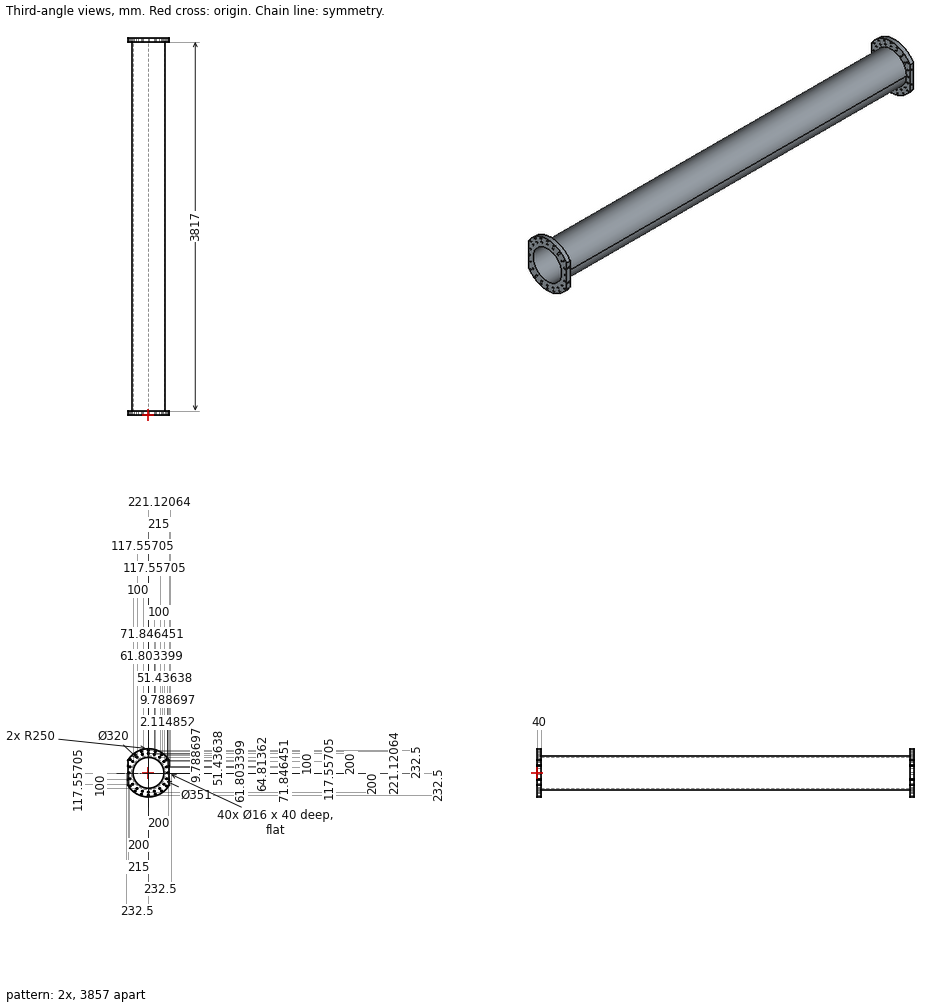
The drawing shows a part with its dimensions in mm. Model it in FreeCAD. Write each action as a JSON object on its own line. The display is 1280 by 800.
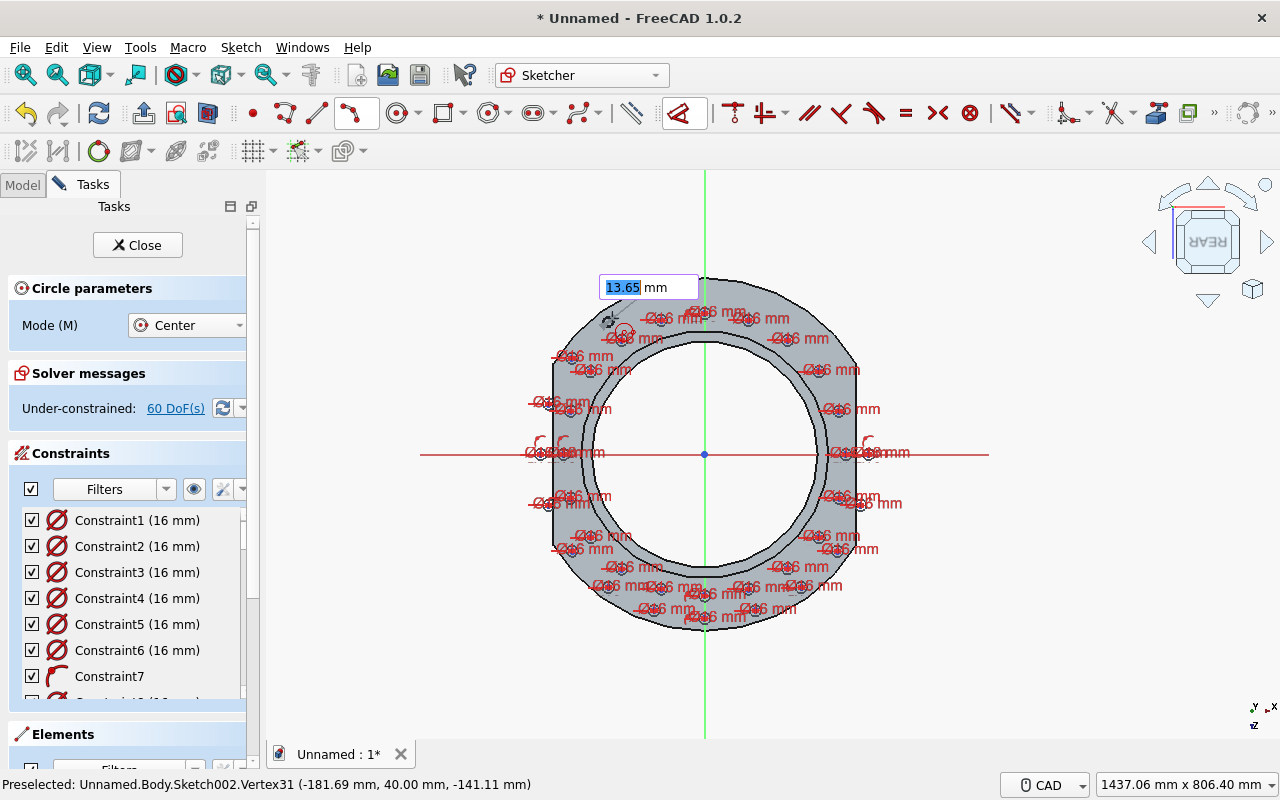
{"action": "type", "text": "16"}
{"action": "key", "text": "Return"}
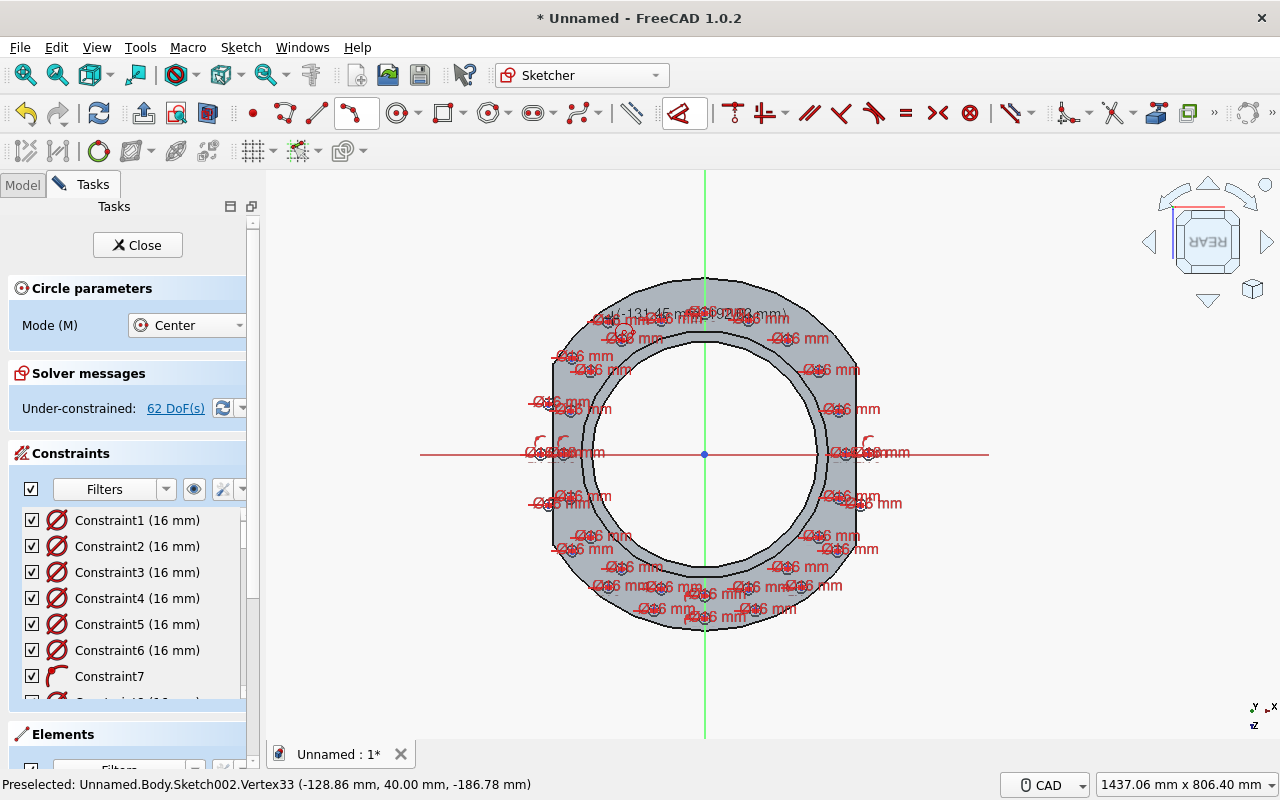
{"action": "scroll", "coordinate": [654, 298], "scroll_direction": "up", "scroll_amount": 7}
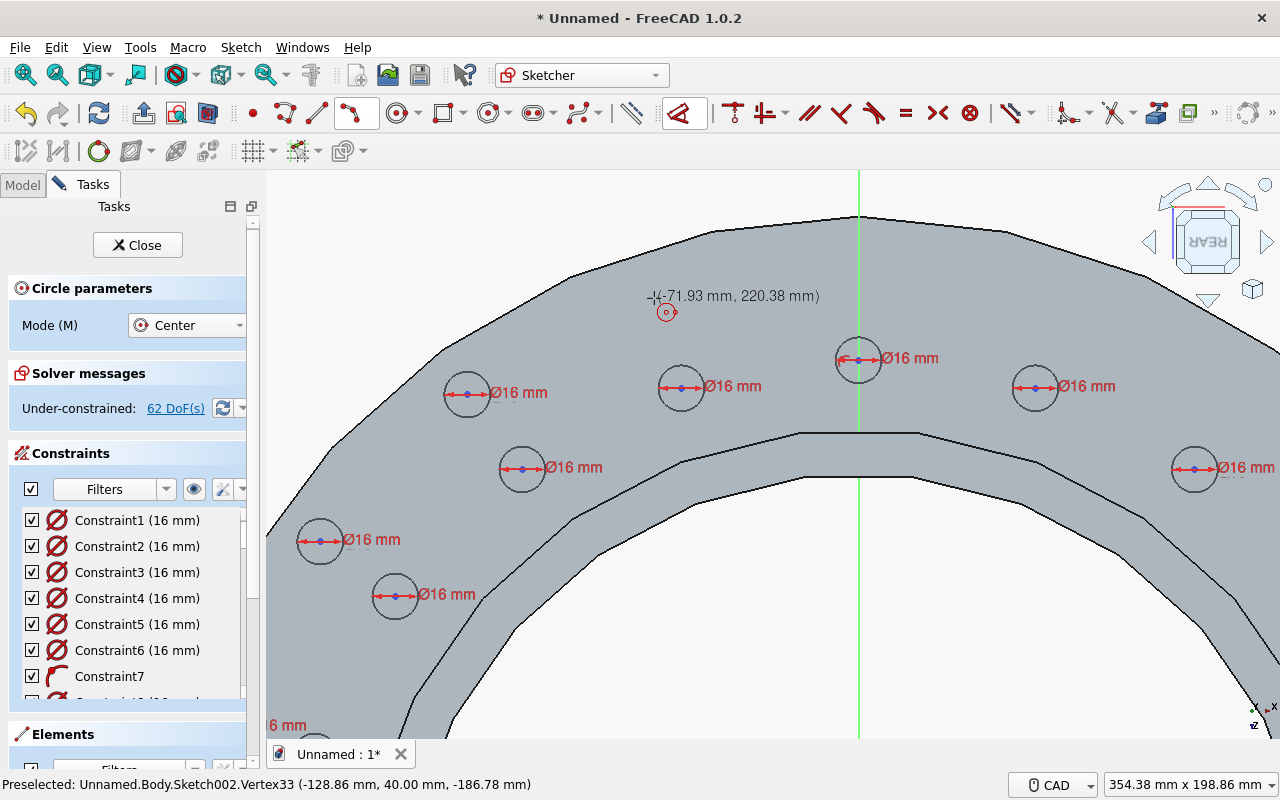
{"action": "left_click", "coordinate": [653, 299]}
{"action": "mouse_move", "coordinate": [669, 283]}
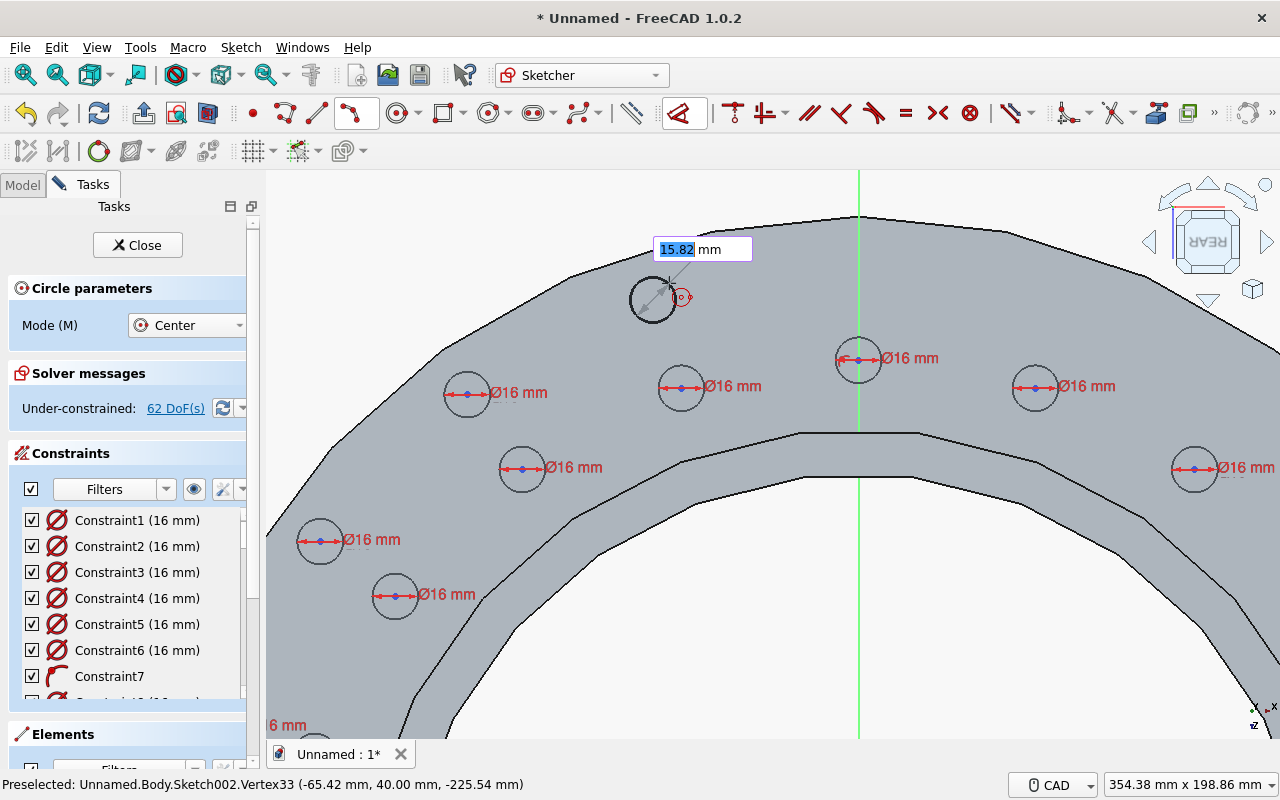
{"action": "type", "text": "16"}
{"action": "key", "text": "Return"}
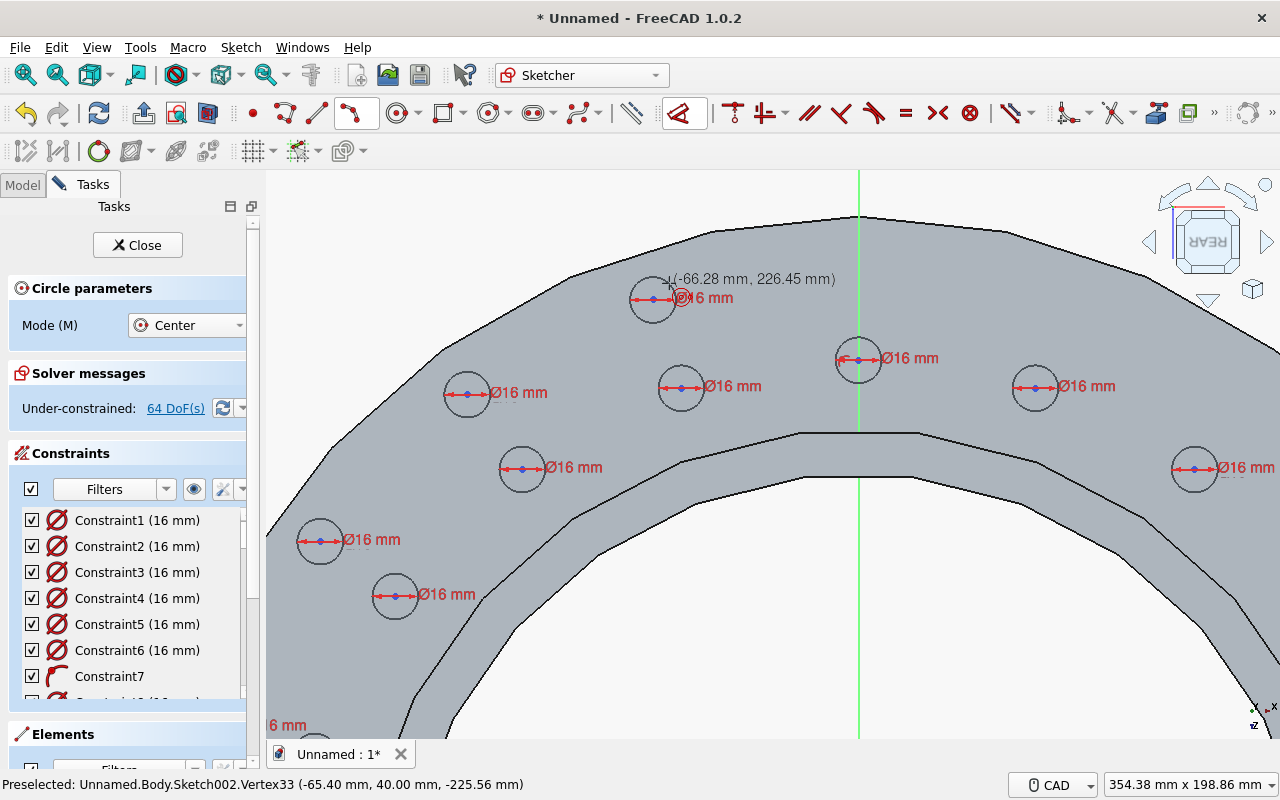
{"action": "left_click", "coordinate": [859, 267]}
{"action": "mouse_move", "coordinate": [875, 250]}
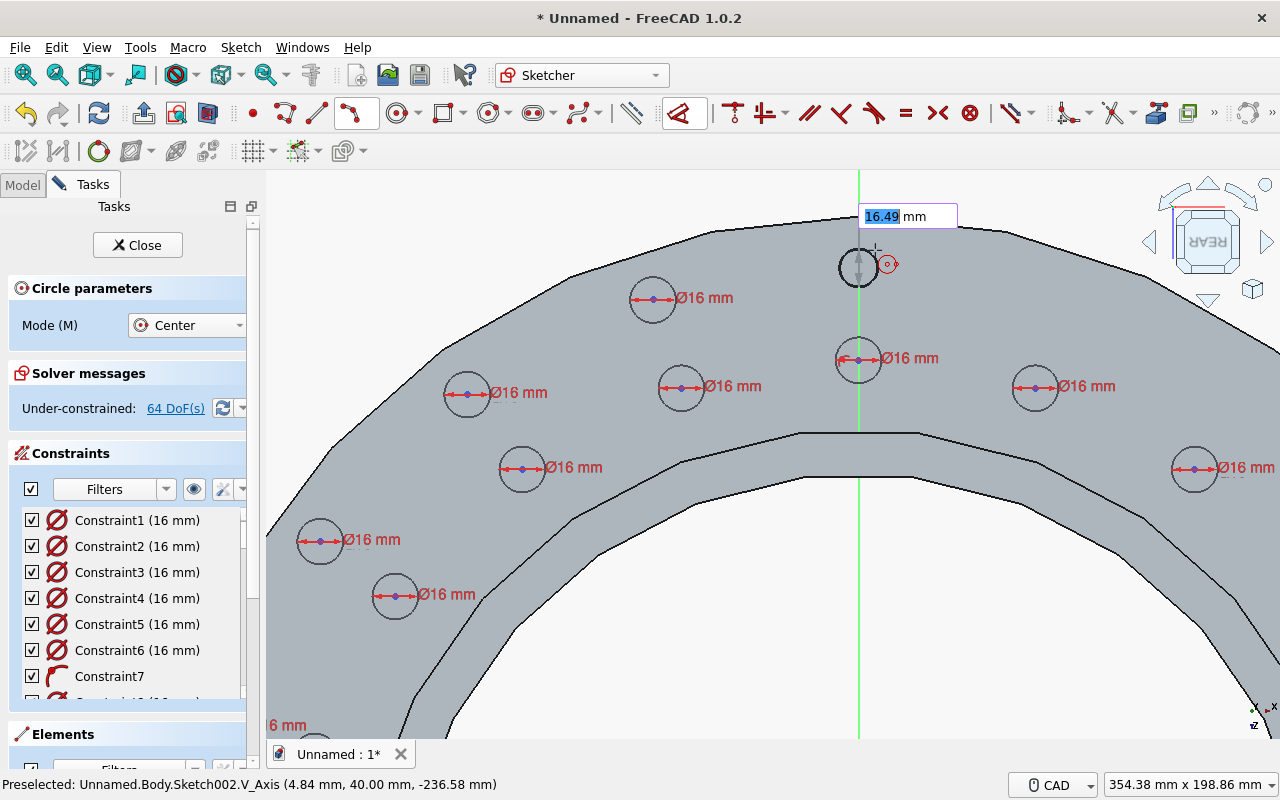
{"action": "type", "text": "16"}
{"action": "key", "text": "Return"}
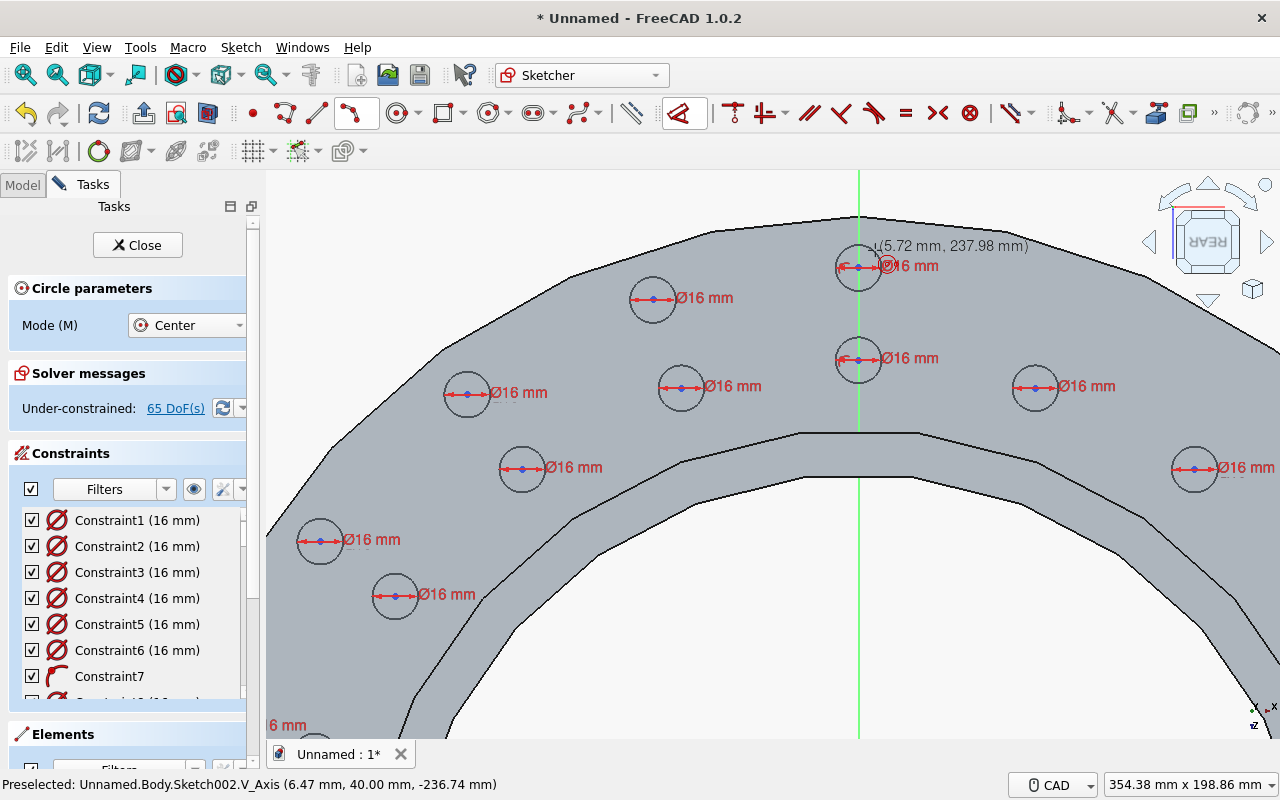
{"action": "left_click", "coordinate": [1064, 299]}
{"action": "mouse_move", "coordinate": [1080, 283]}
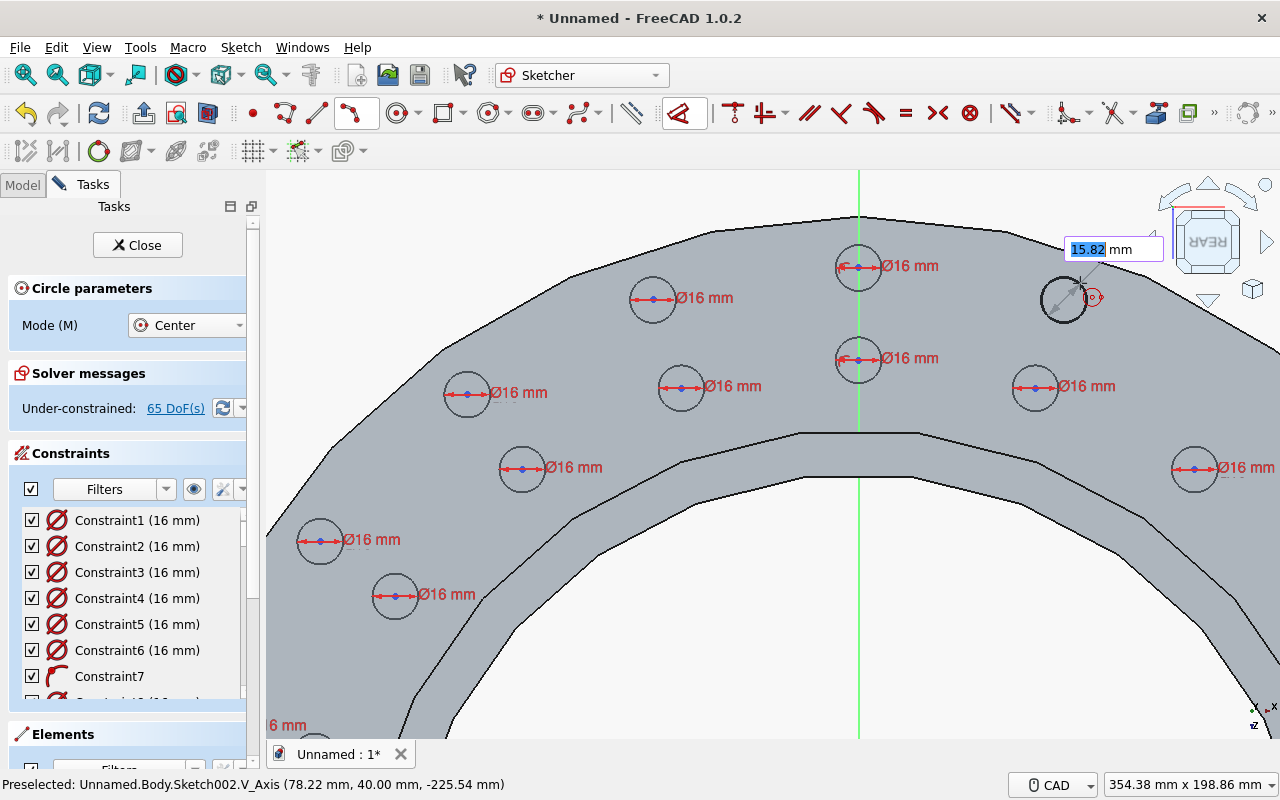
{"action": "type", "text": "16"}
{"action": "key", "text": "Return"}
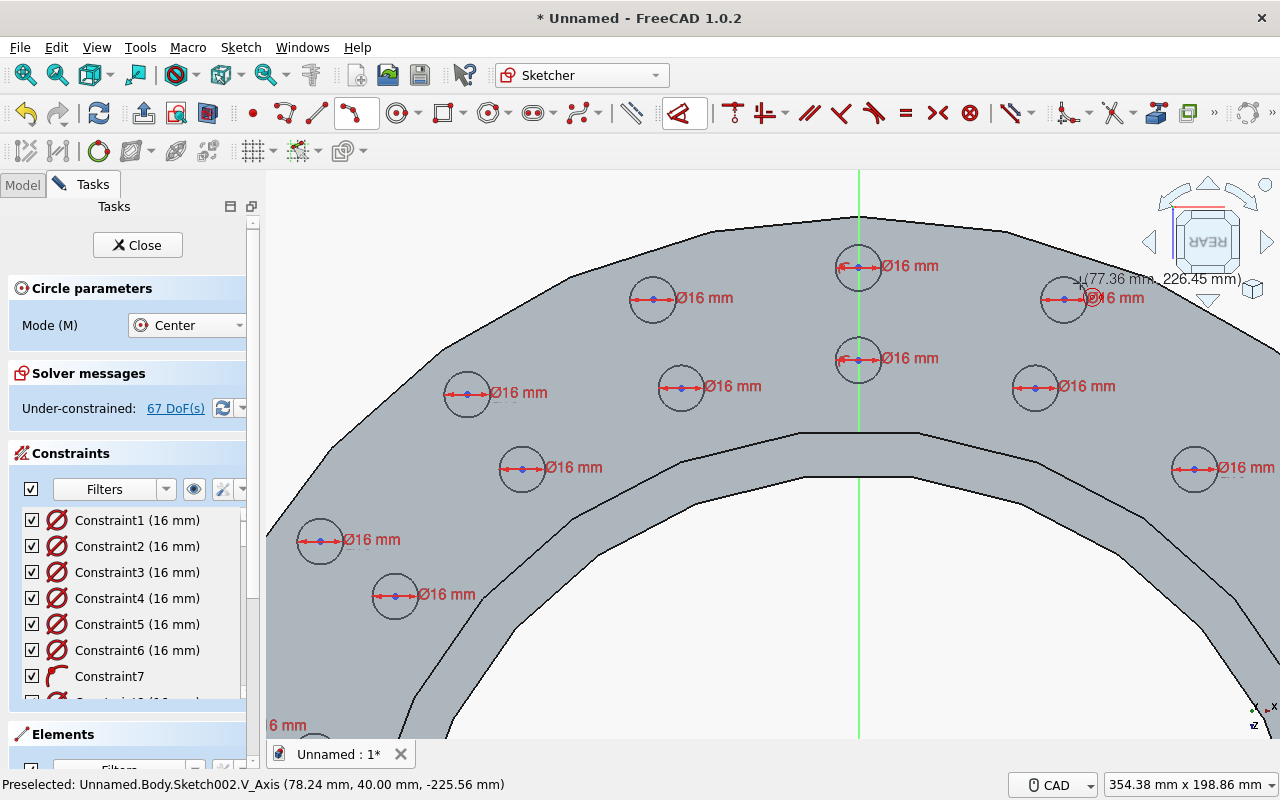
{"action": "scroll", "coordinate": [654, 298], "scroll_direction": "down", "scroll_amount": 7}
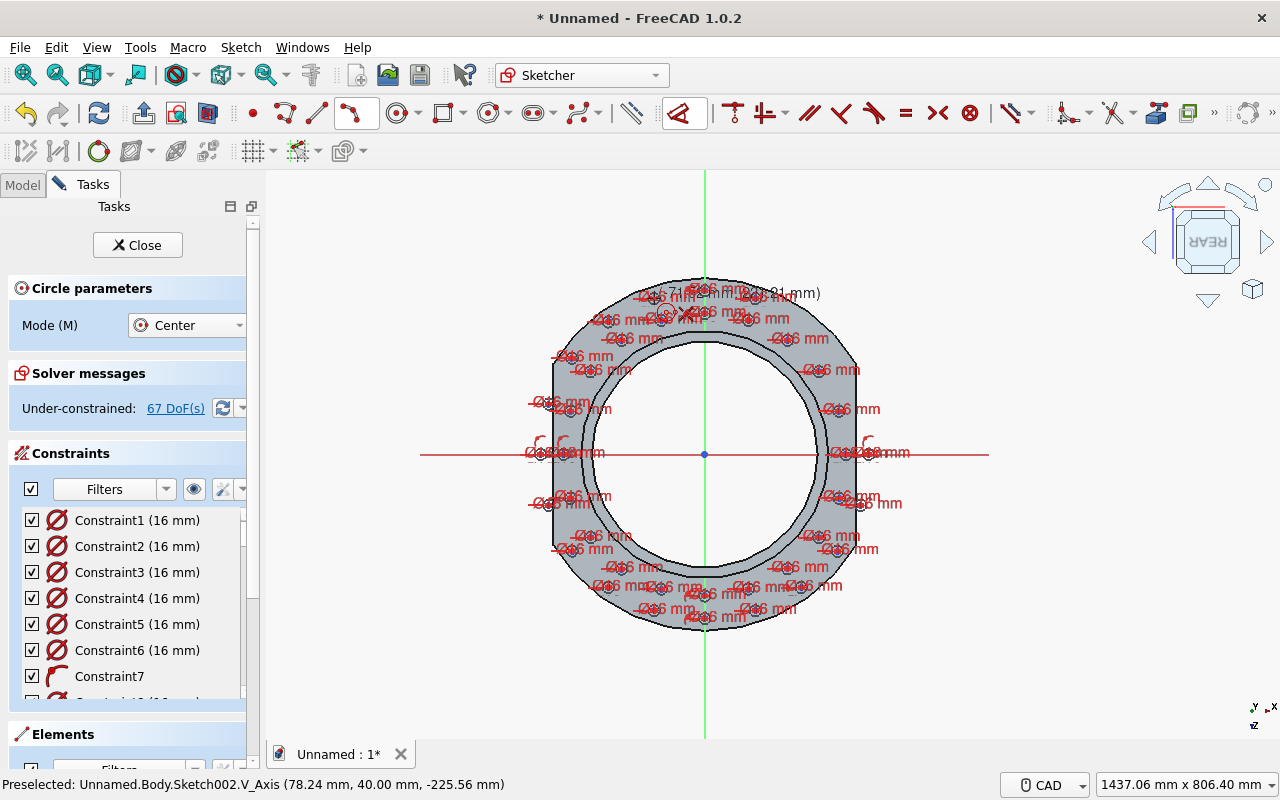
{"action": "scroll", "coordinate": [801, 322], "scroll_direction": "up", "scroll_amount": 7}